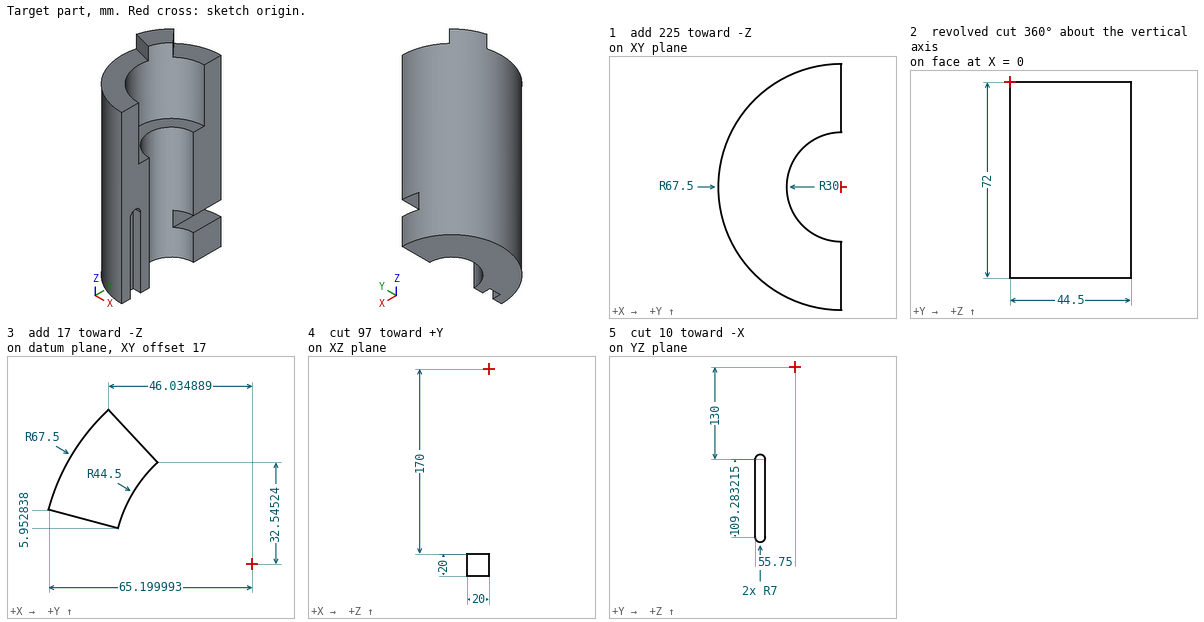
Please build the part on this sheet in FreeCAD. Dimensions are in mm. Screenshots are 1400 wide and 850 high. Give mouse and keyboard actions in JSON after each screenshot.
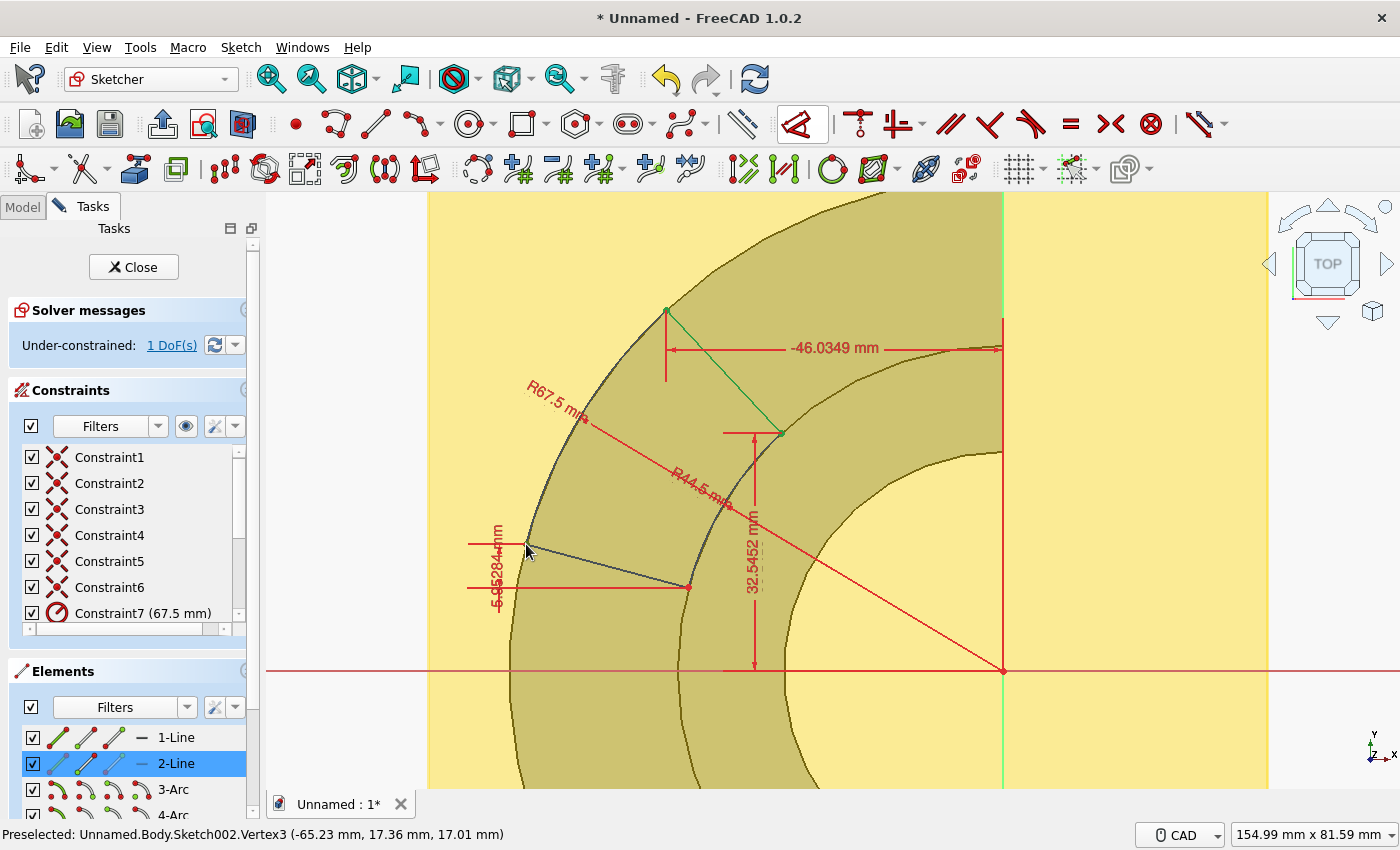
{"action": "key", "text": "l"}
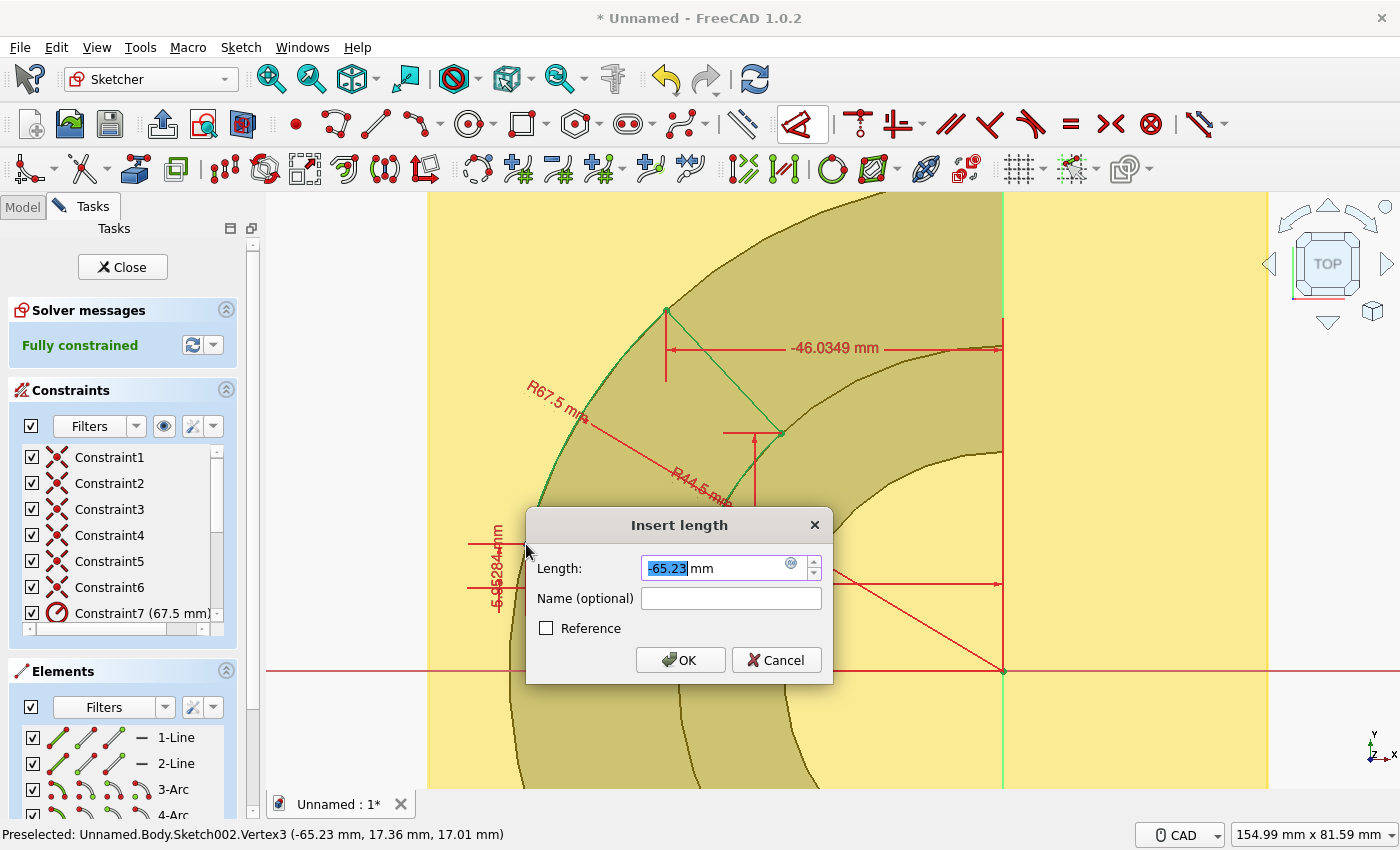
{"action": "type", "text": "-65.199993"}
{"action": "key", "text": "Return"}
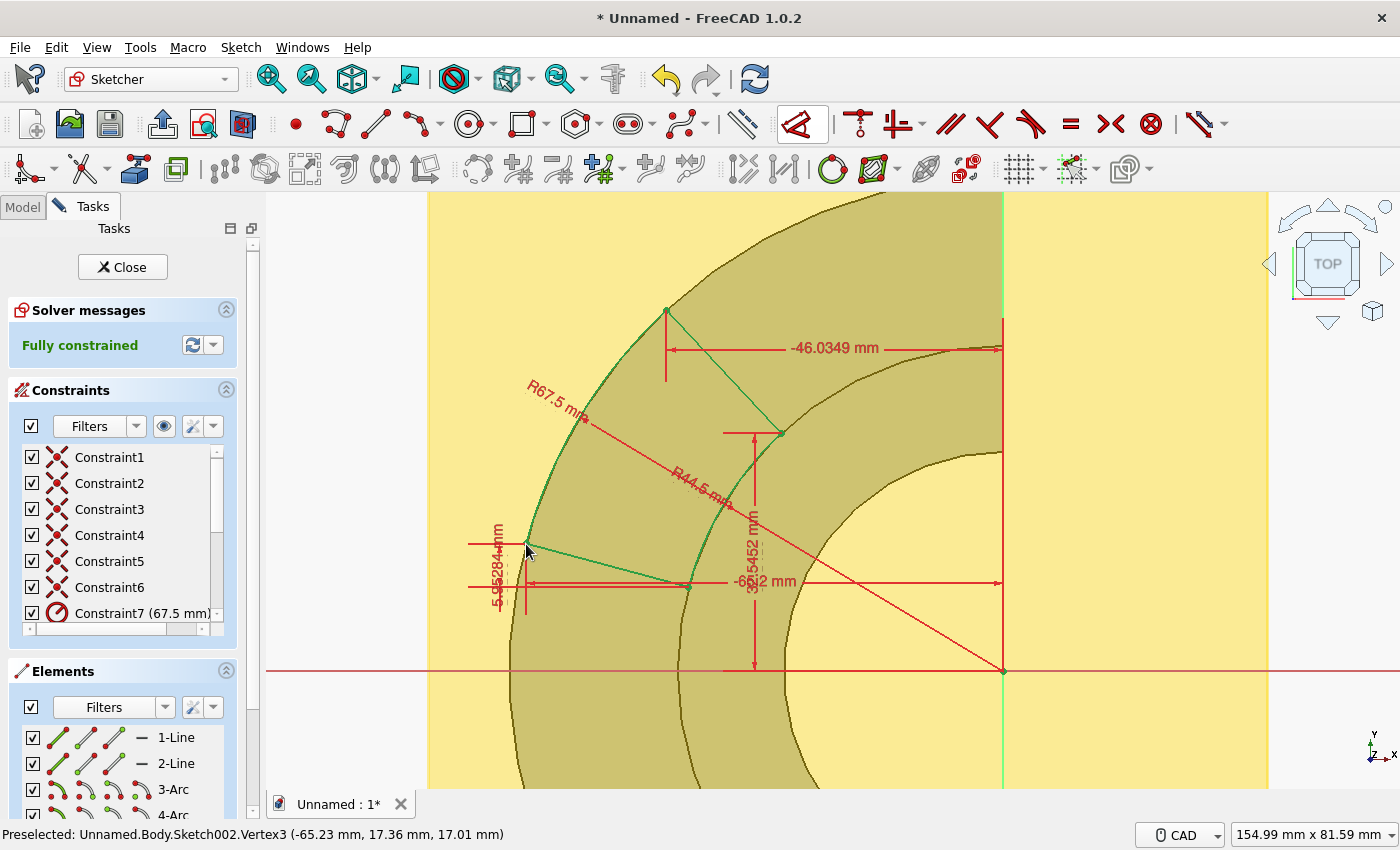
{"action": "left_click", "coordinate": [123, 267]}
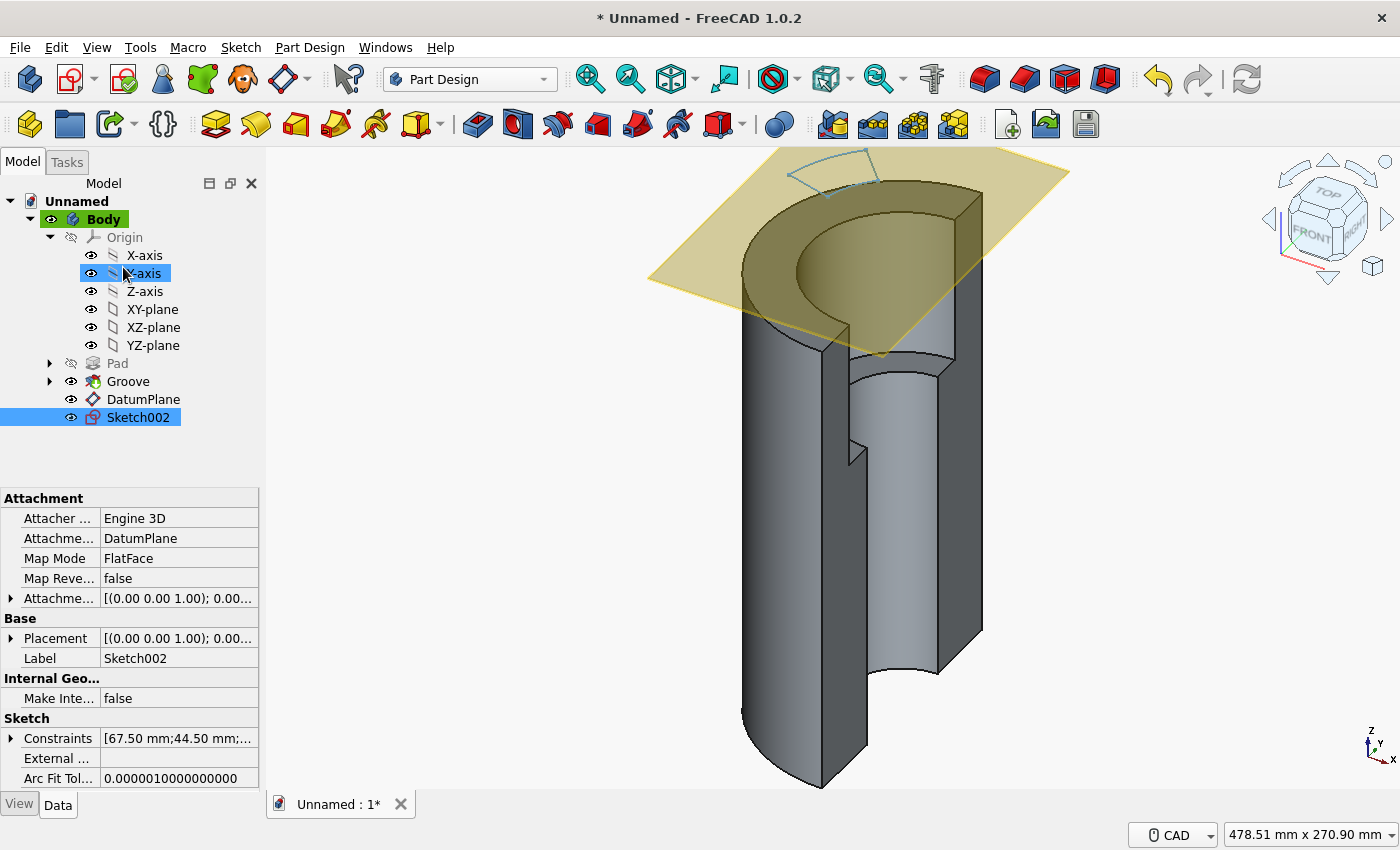
{"action": "left_click", "coordinate": [216, 124]}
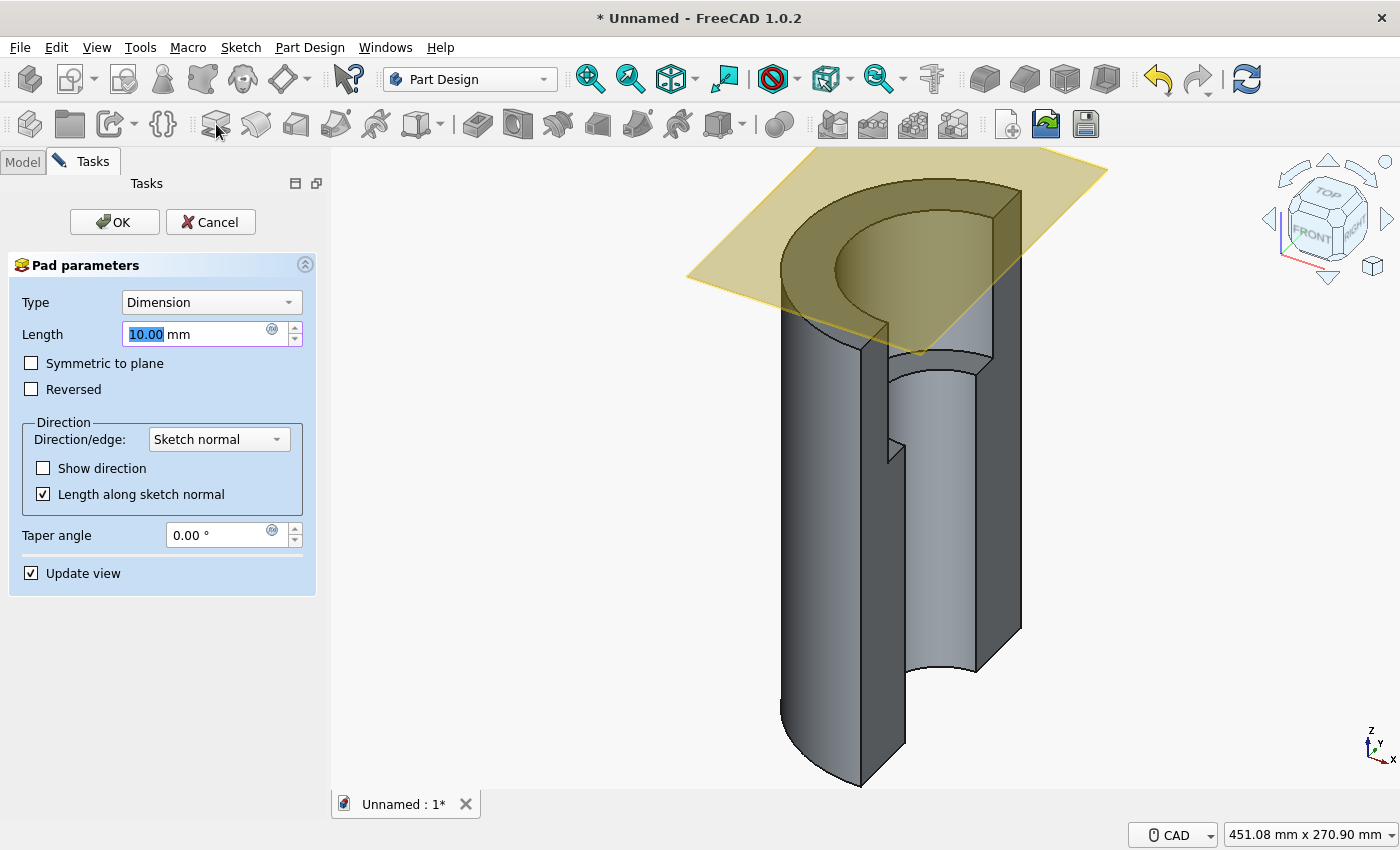
{"action": "type", "text": "17"}
{"action": "key", "text": "Tab"}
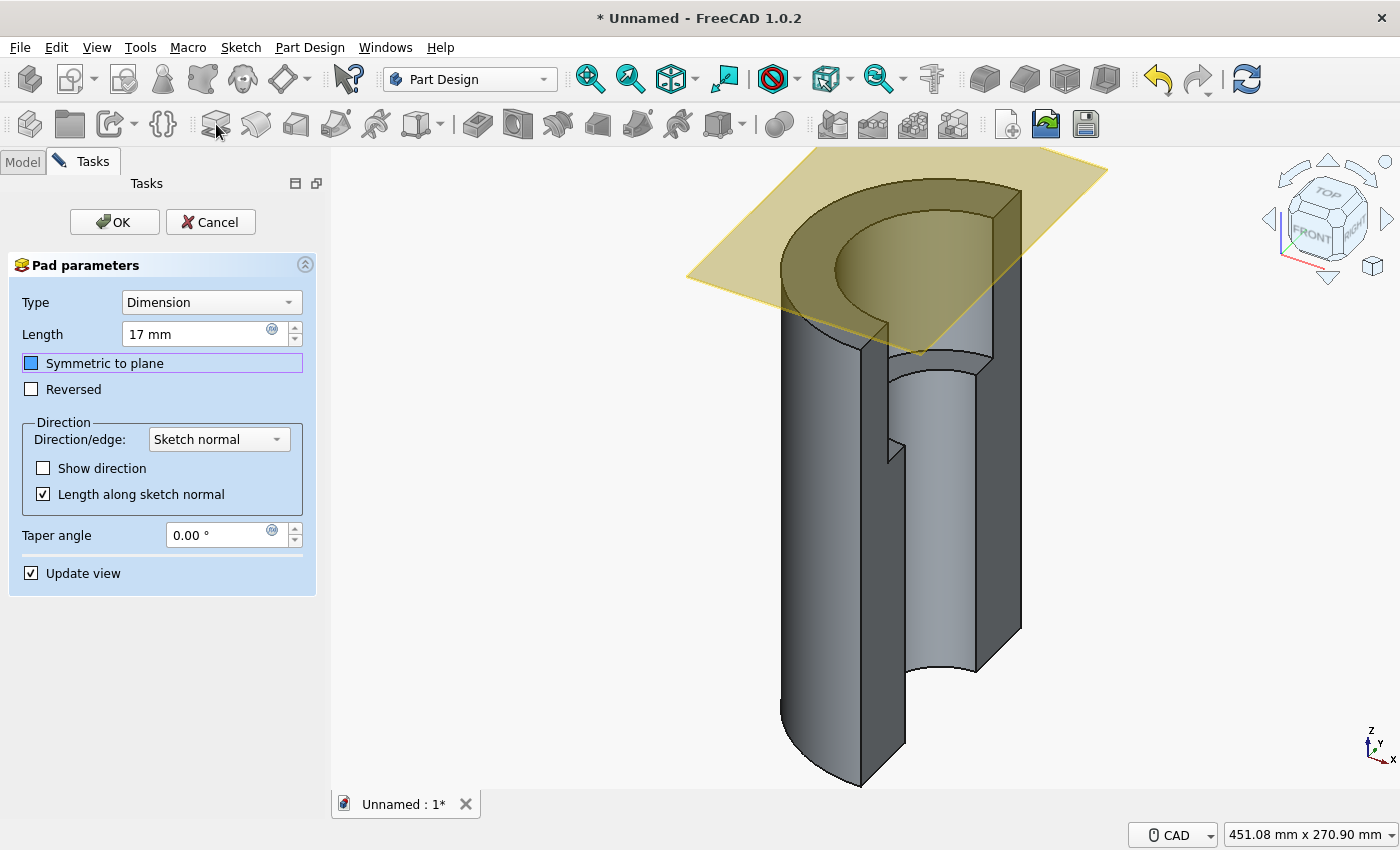
{"action": "left_click", "coordinate": [30, 389]}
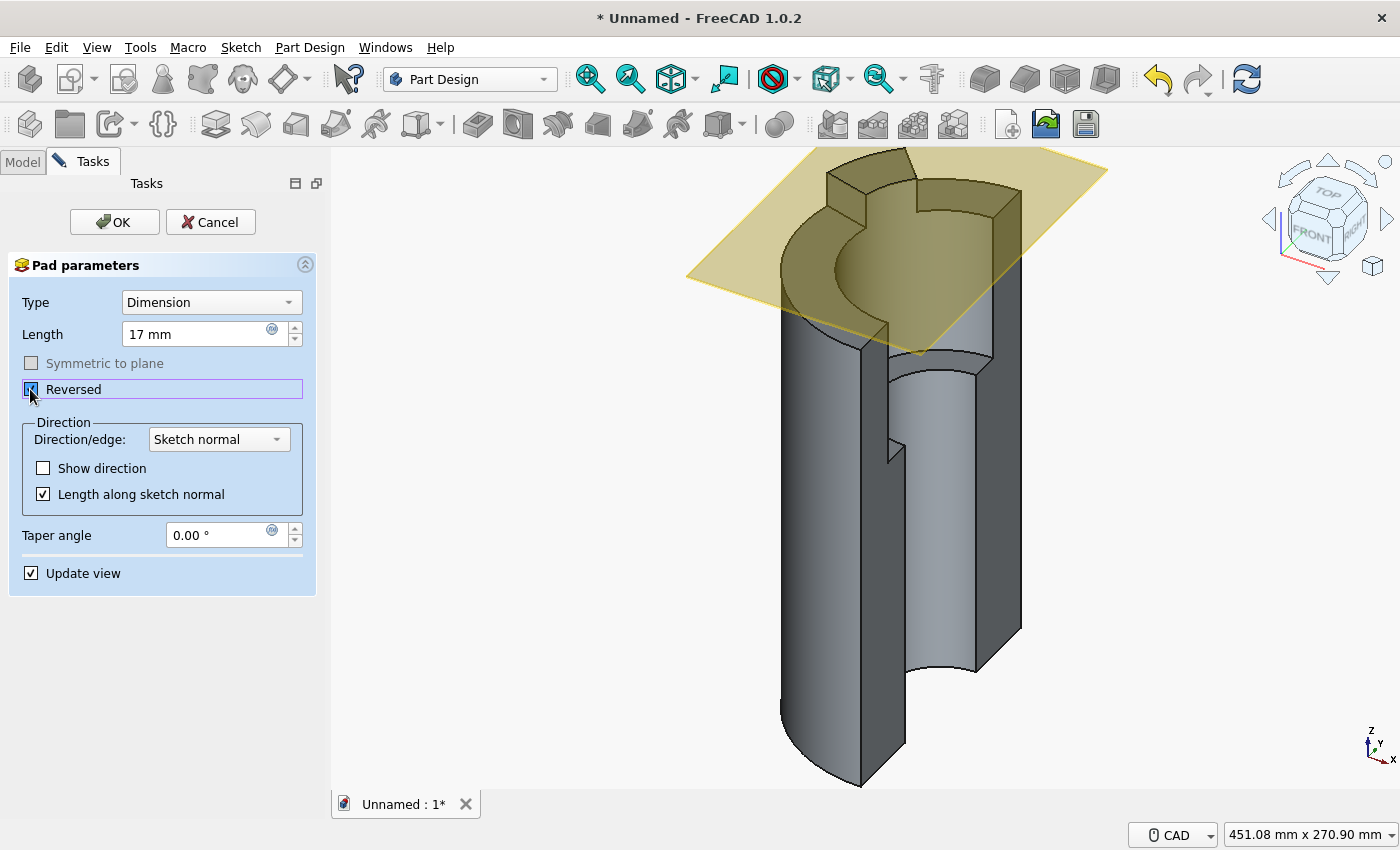
{"action": "left_click", "coordinate": [115, 222]}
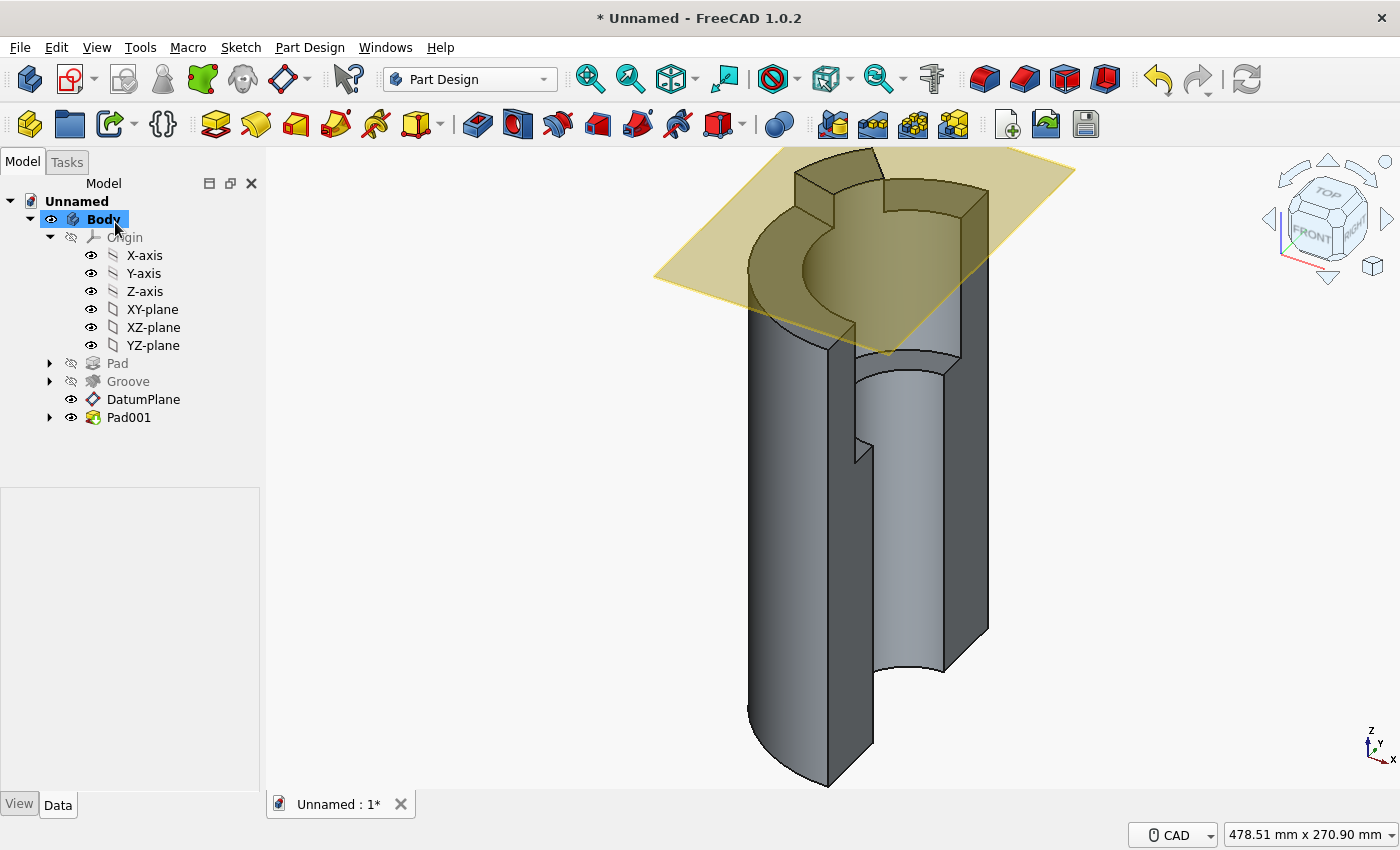
{"action": "left_click", "coordinate": [116, 399]}
{"action": "key", "text": "space"}